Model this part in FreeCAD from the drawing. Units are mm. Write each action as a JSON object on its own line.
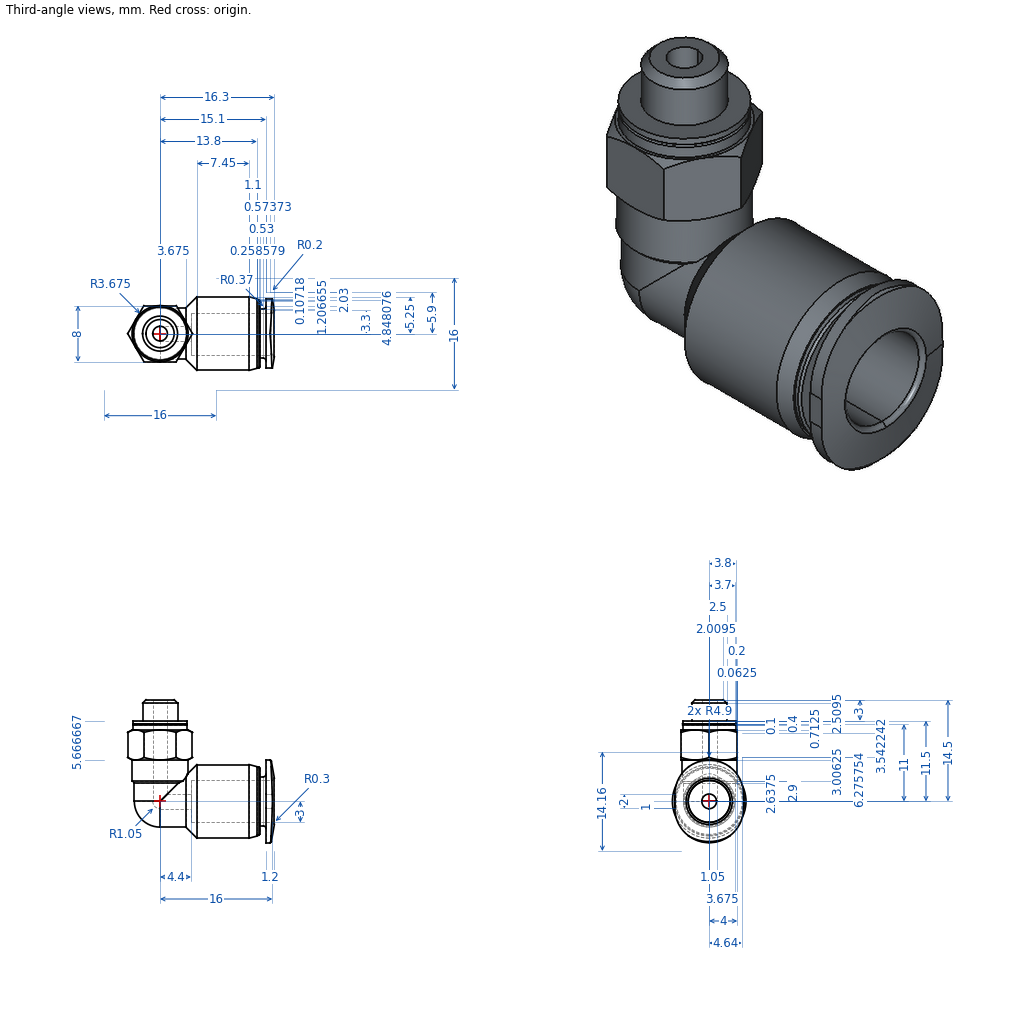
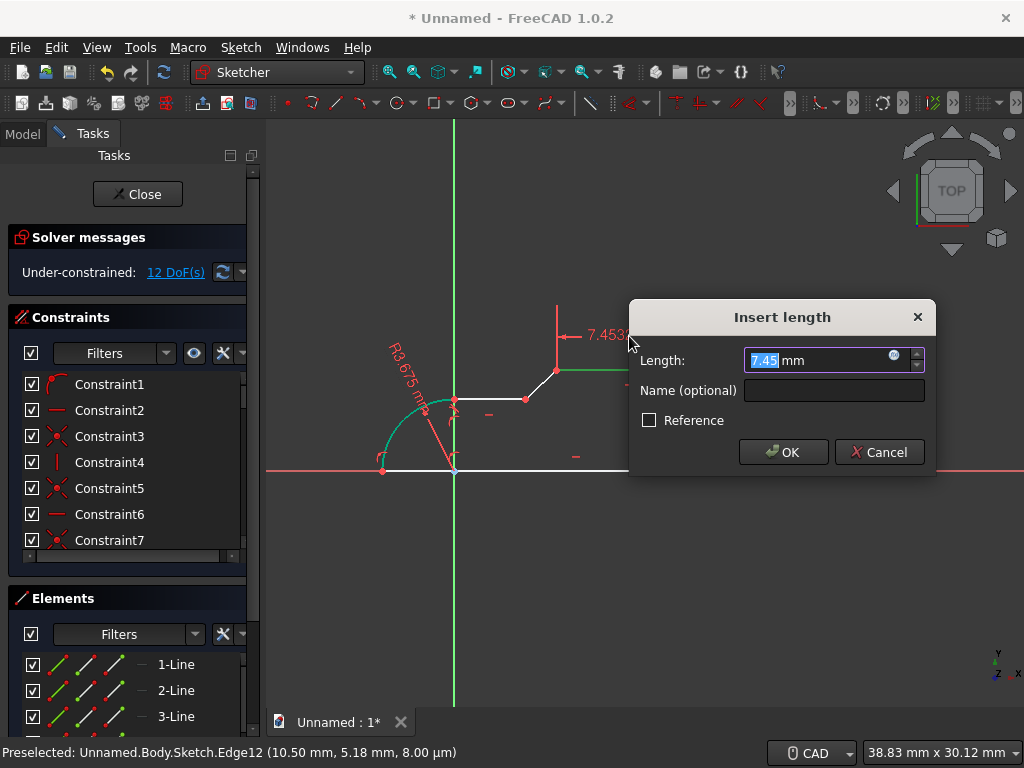
{"action": "type", "text": "7.45"}
{"action": "key", "text": "Return"}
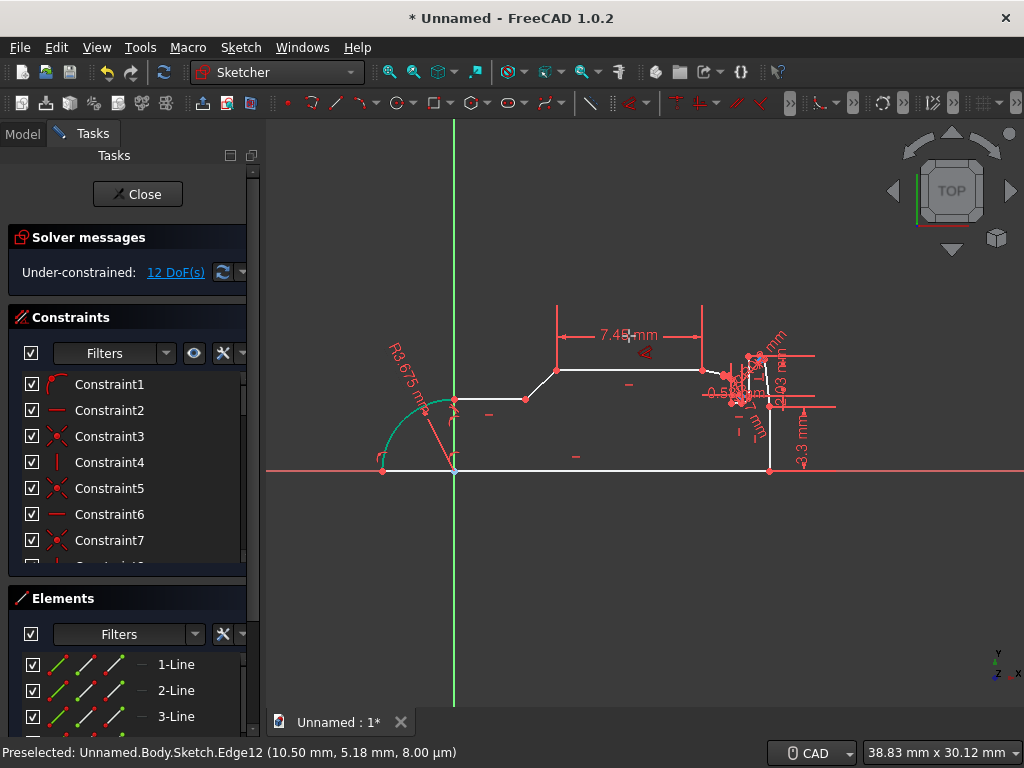
{"action": "scroll", "coordinate": [761, 356], "scroll_direction": "up", "scroll_amount": 6}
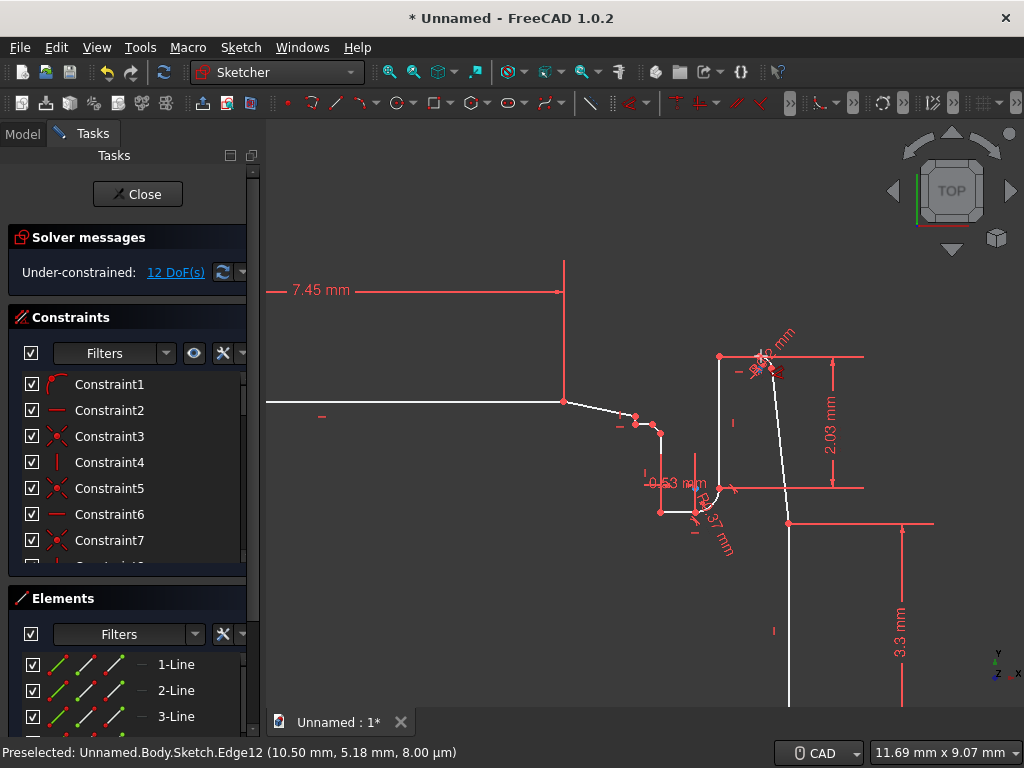
{"action": "left_click", "coordinate": [759, 357]}
{"action": "left_click", "coordinate": [817, 518]}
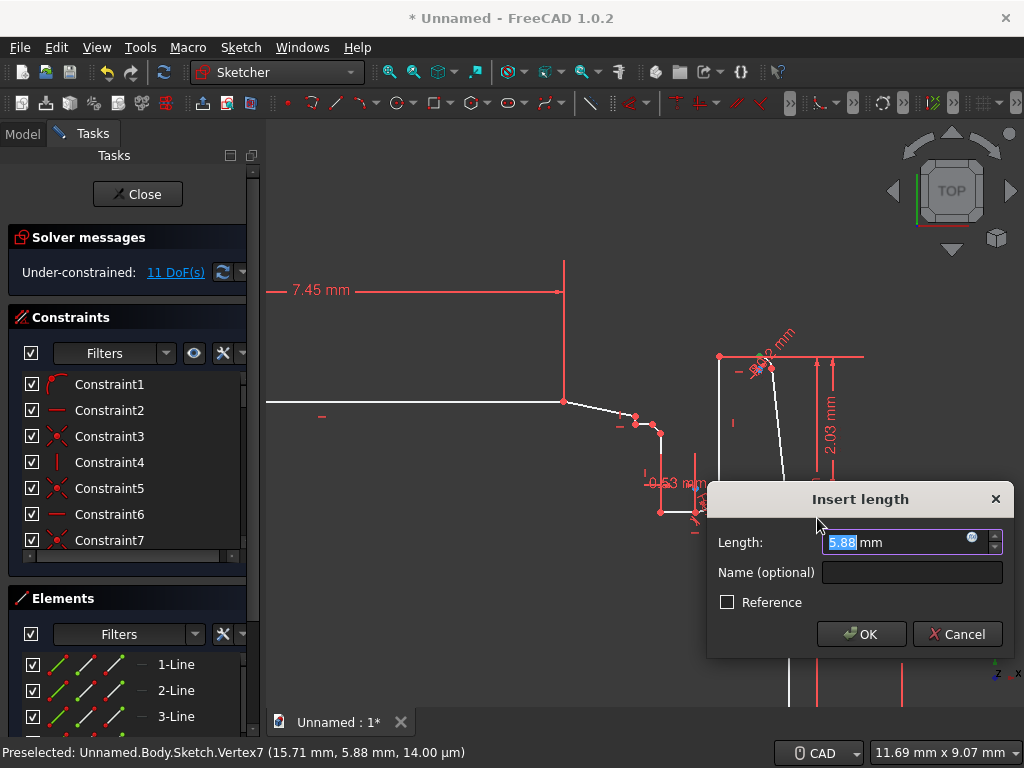
{"action": "type", "text": "5.9"}
{"action": "key", "text": "Return"}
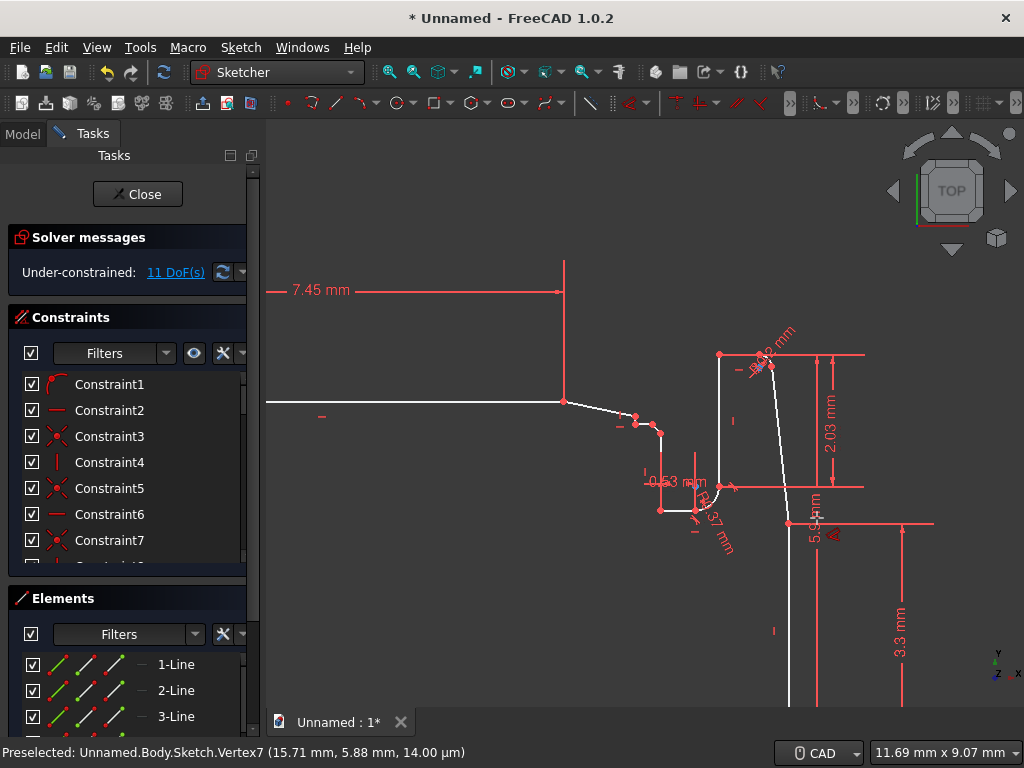
{"action": "left_click", "coordinate": [614, 412]}
{"action": "left_click", "coordinate": [600, 368]}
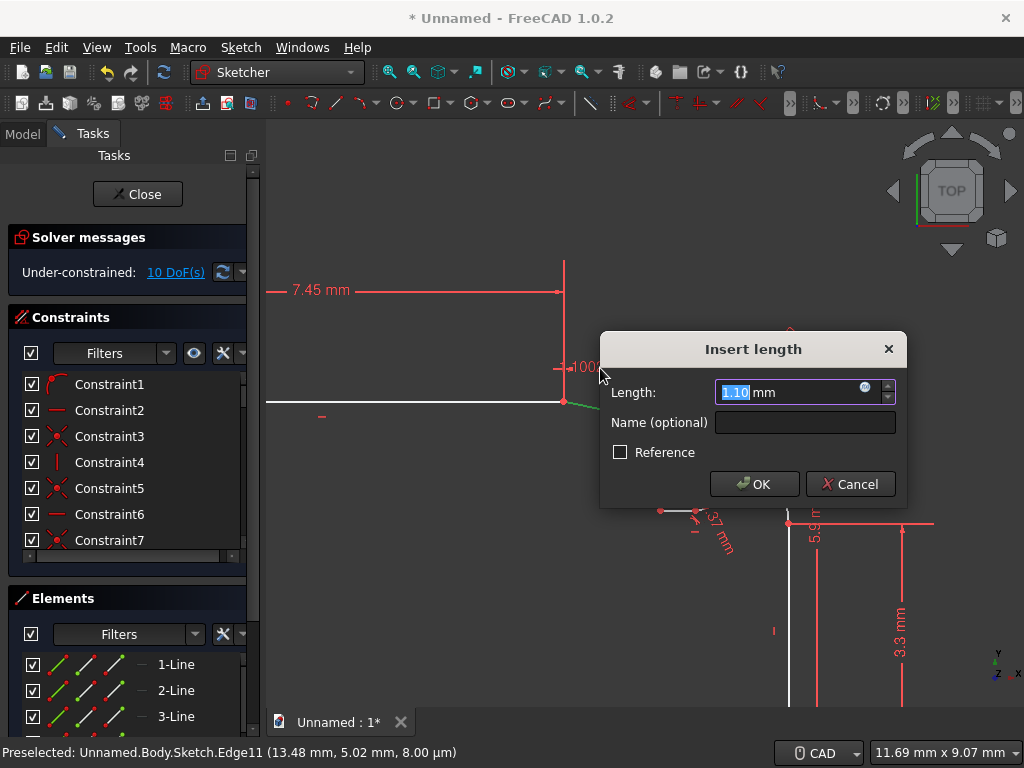
{"action": "type", "text": "1.1"}
{"action": "key", "text": "Return"}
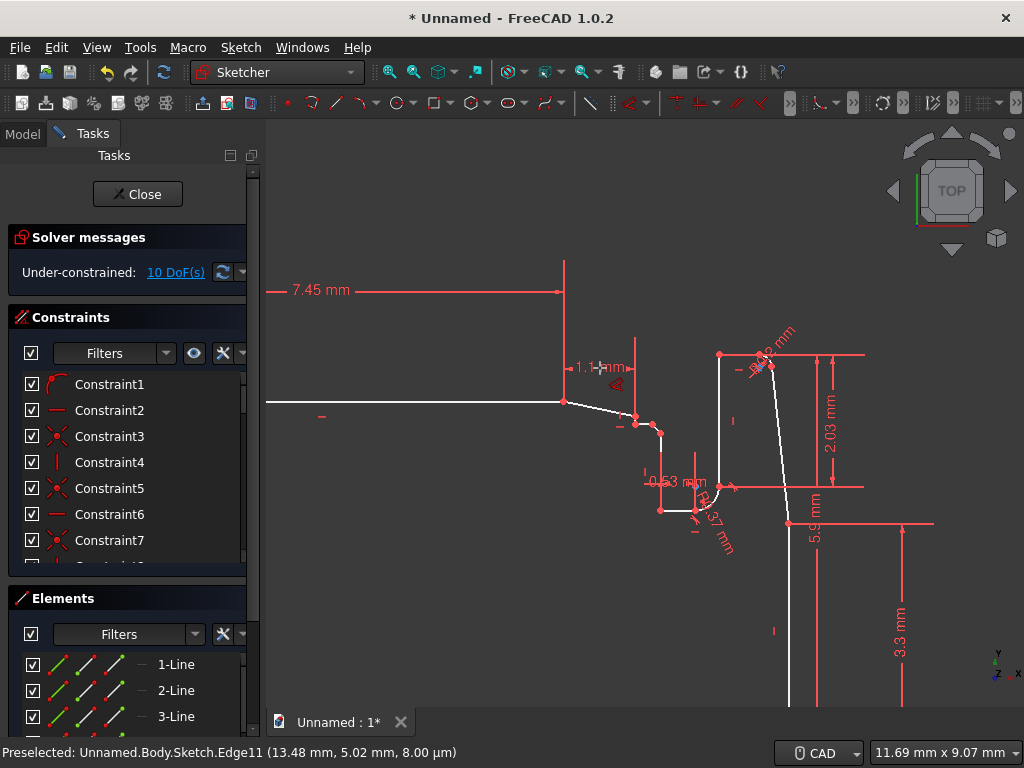
{"action": "scroll", "coordinate": [760, 356], "scroll_direction": "down", "scroll_amount": 6}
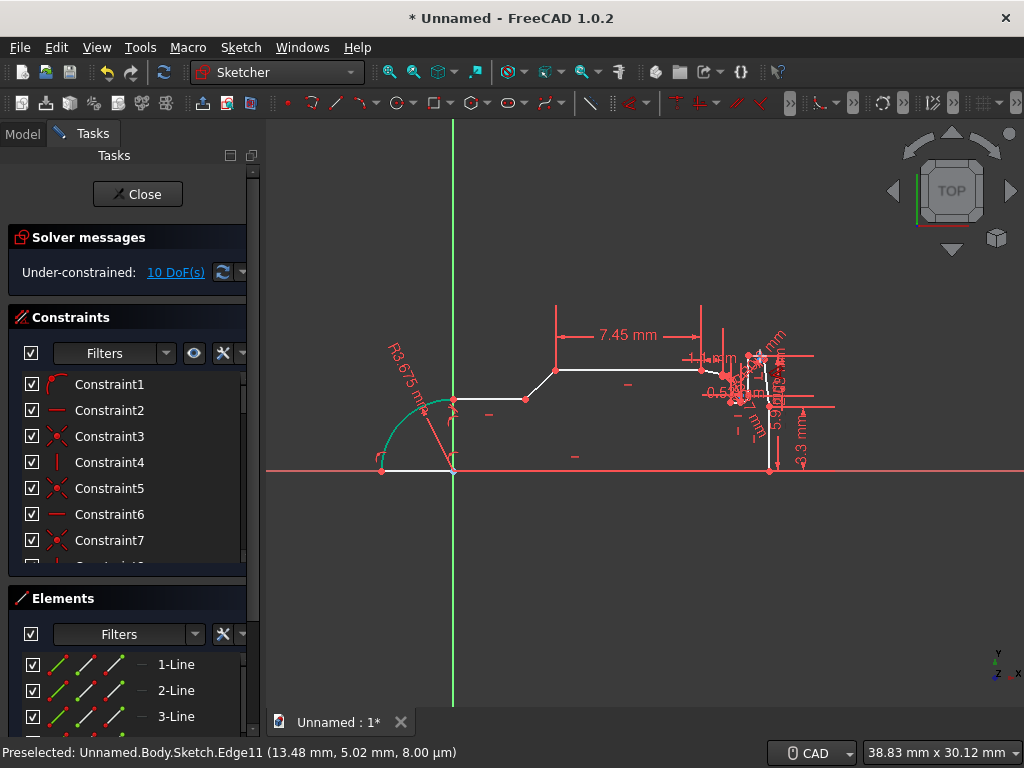
{"action": "left_click", "coordinate": [504, 399]}
{"action": "left_click", "coordinate": [489, 365]}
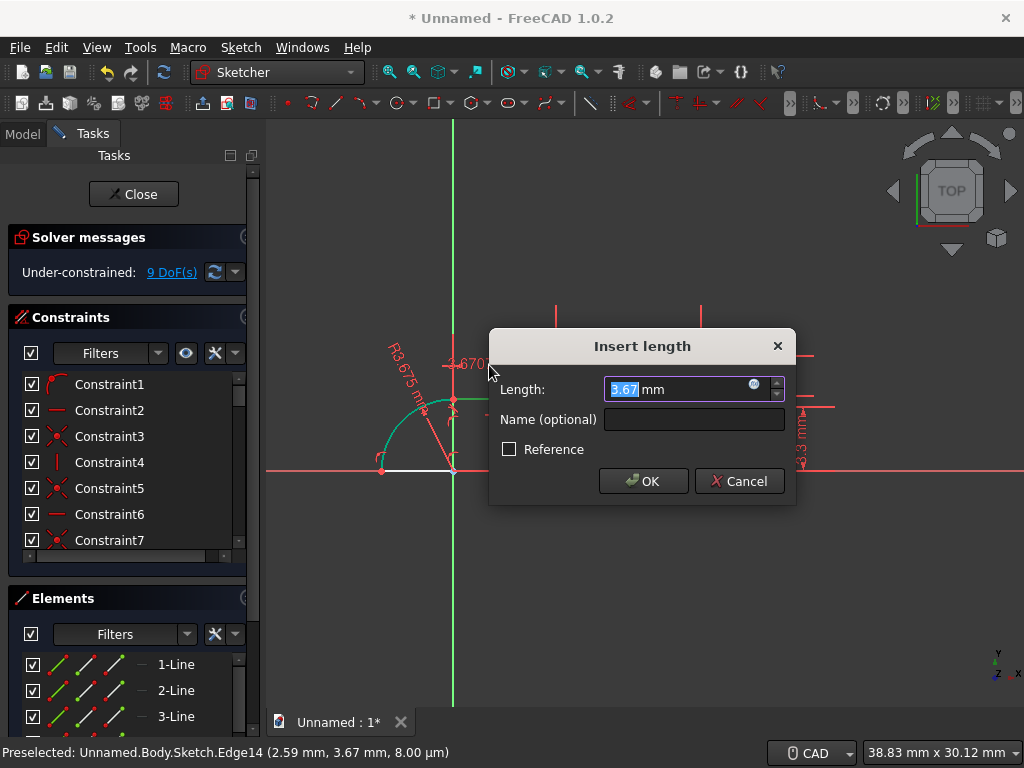
{"action": "type", "text": "3.675"}
{"action": "key", "text": "Return"}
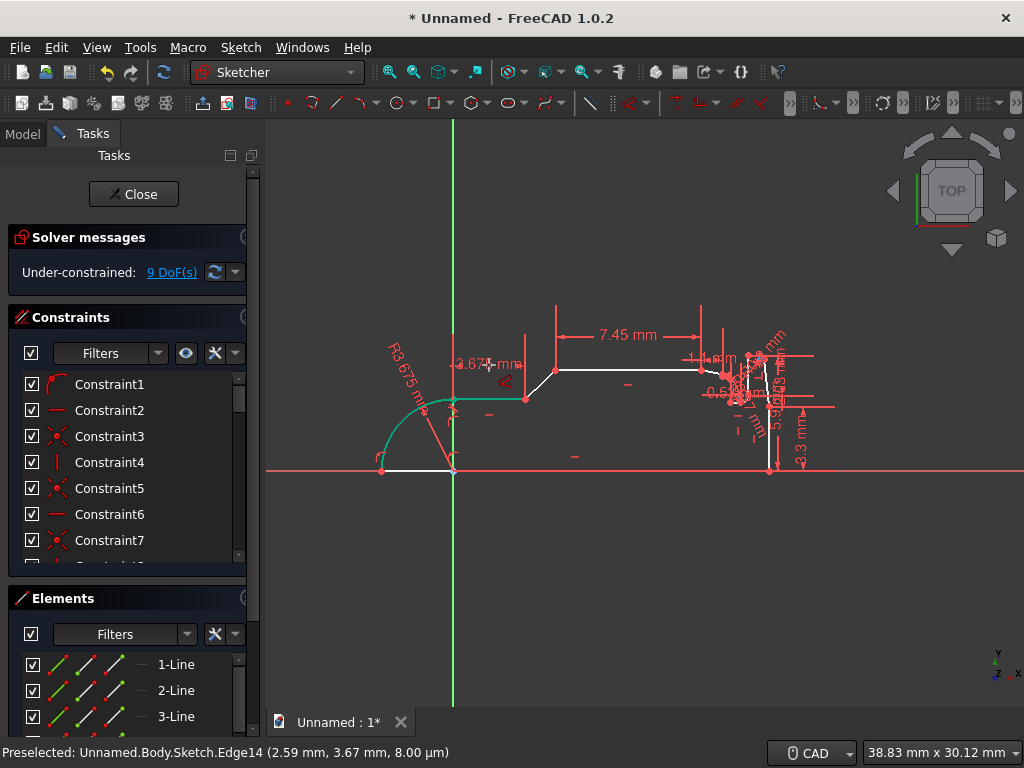
{"action": "left_click", "coordinate": [769, 471]}
{"action": "left_click", "coordinate": [611, 505]}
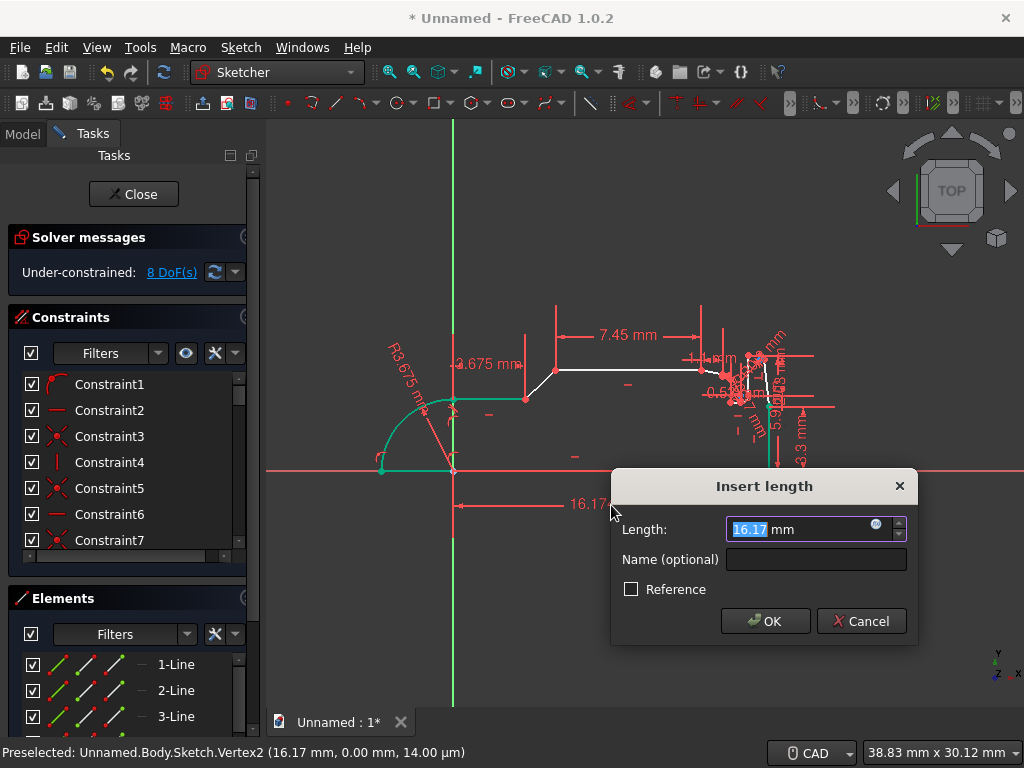
{"action": "type", "text": "16.3"}
{"action": "key", "text": "Return"}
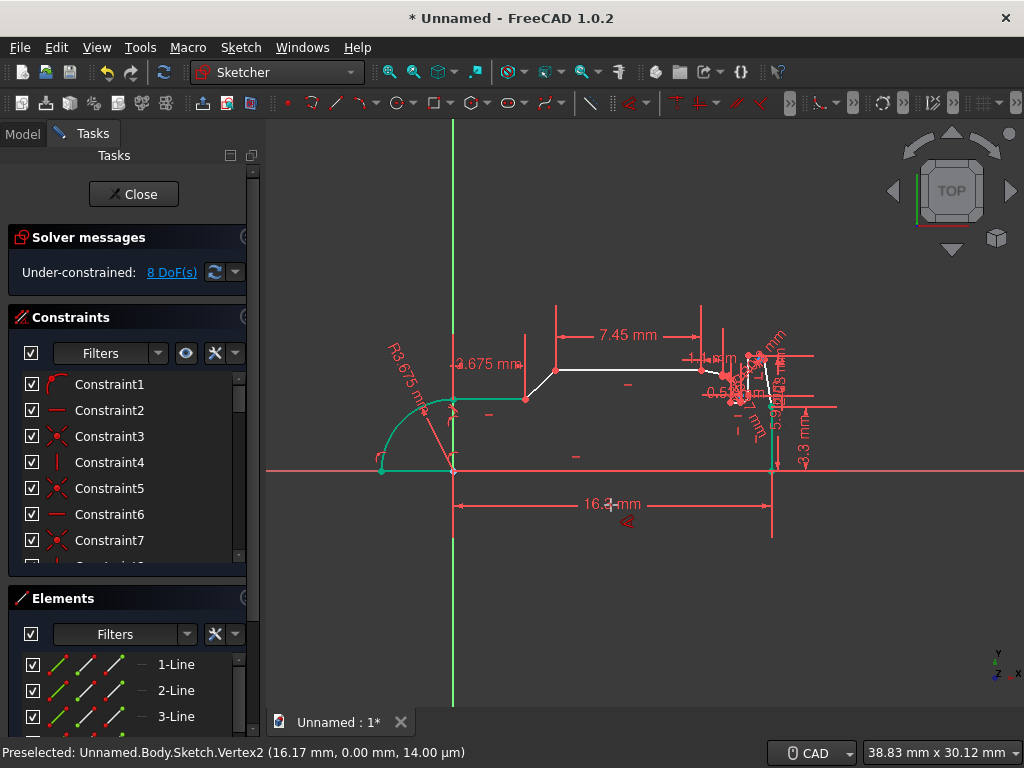
{"action": "left_click", "coordinate": [748, 356]}
{"action": "left_click", "coordinate": [533, 322]}